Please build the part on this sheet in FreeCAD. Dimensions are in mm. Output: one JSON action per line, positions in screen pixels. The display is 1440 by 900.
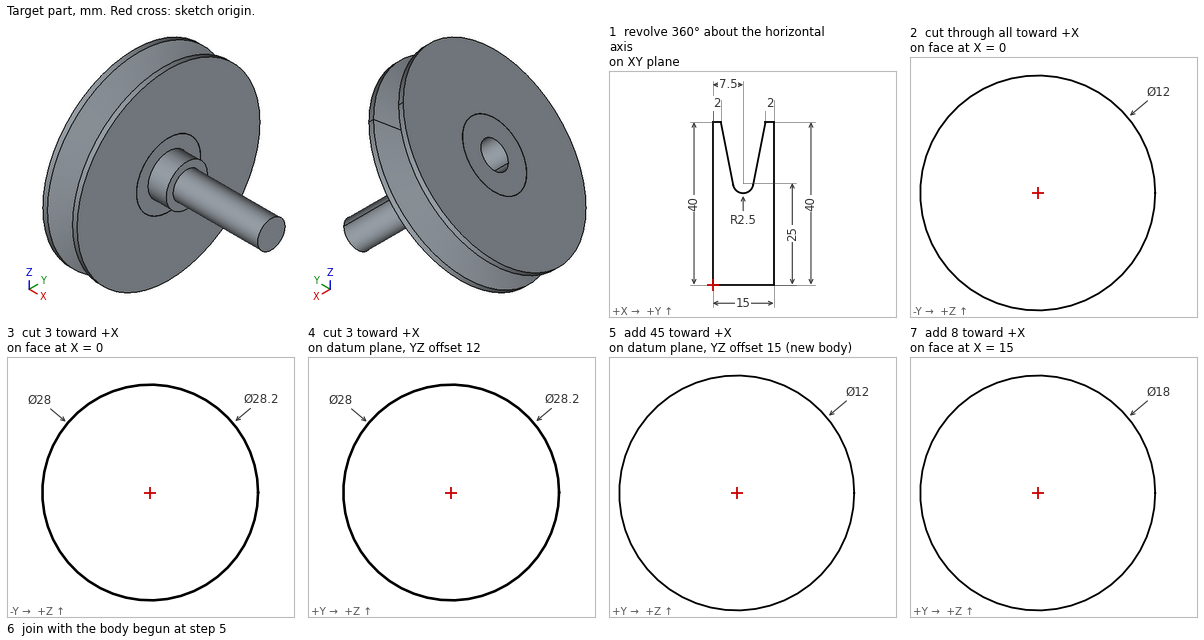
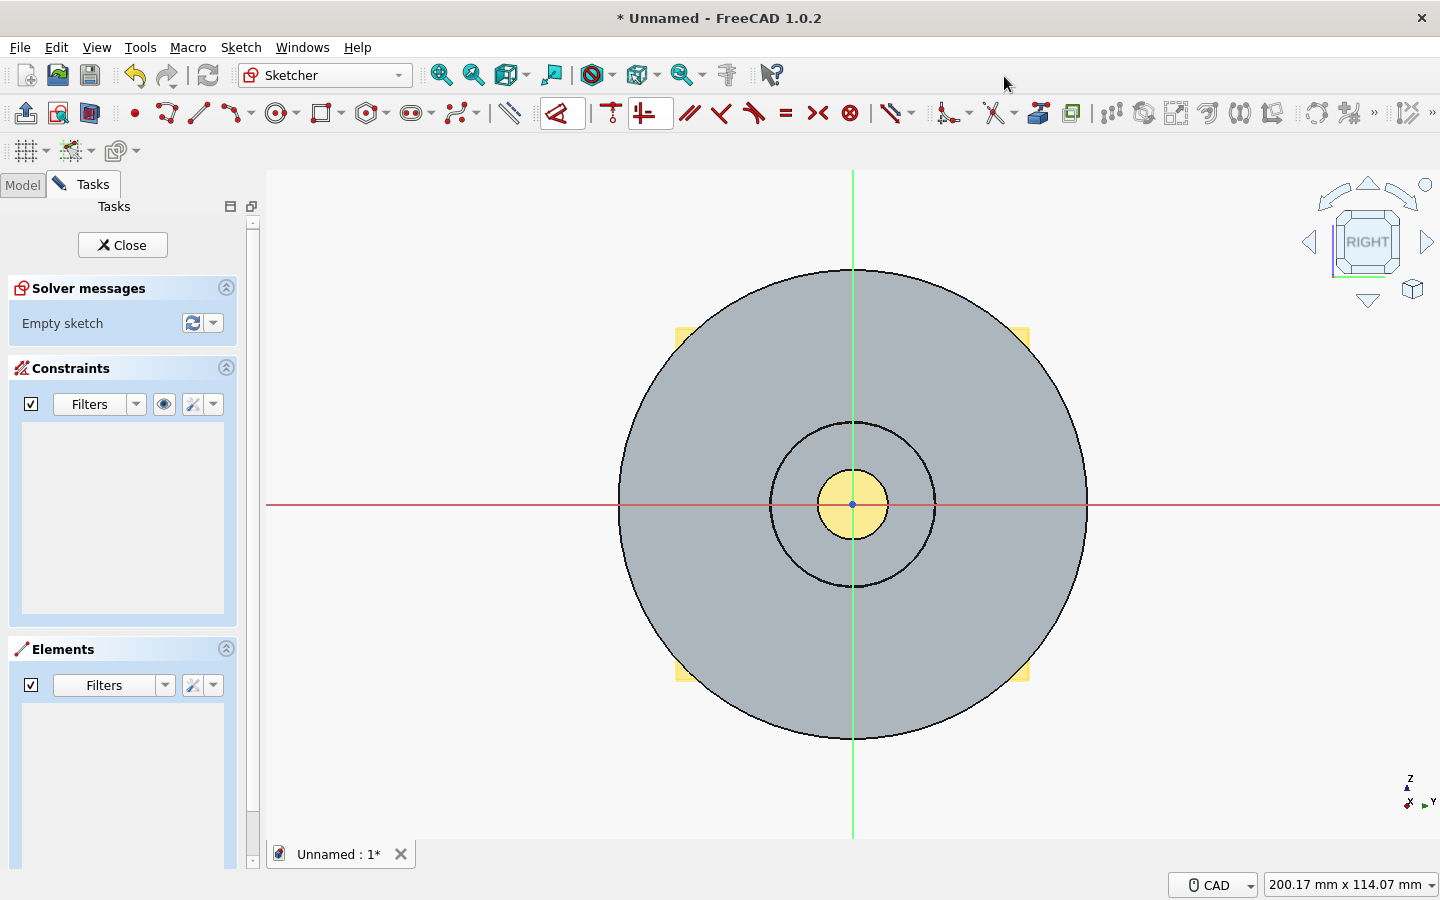
{"action": "scroll", "coordinate": [866, 505], "scroll_direction": "up", "scroll_amount": 9}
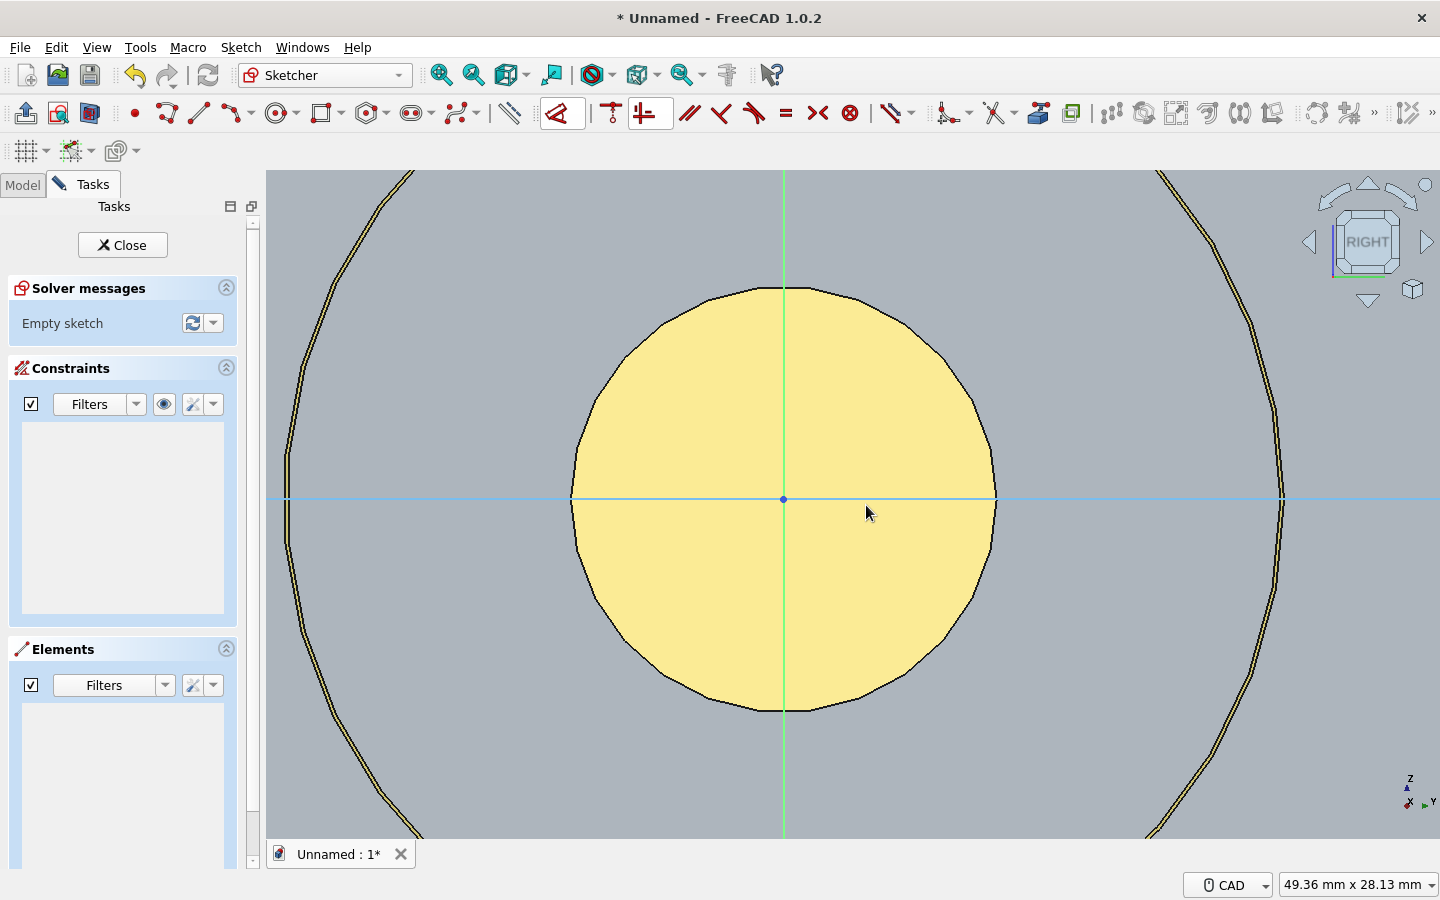
{"action": "left_click", "coordinate": [276, 114]}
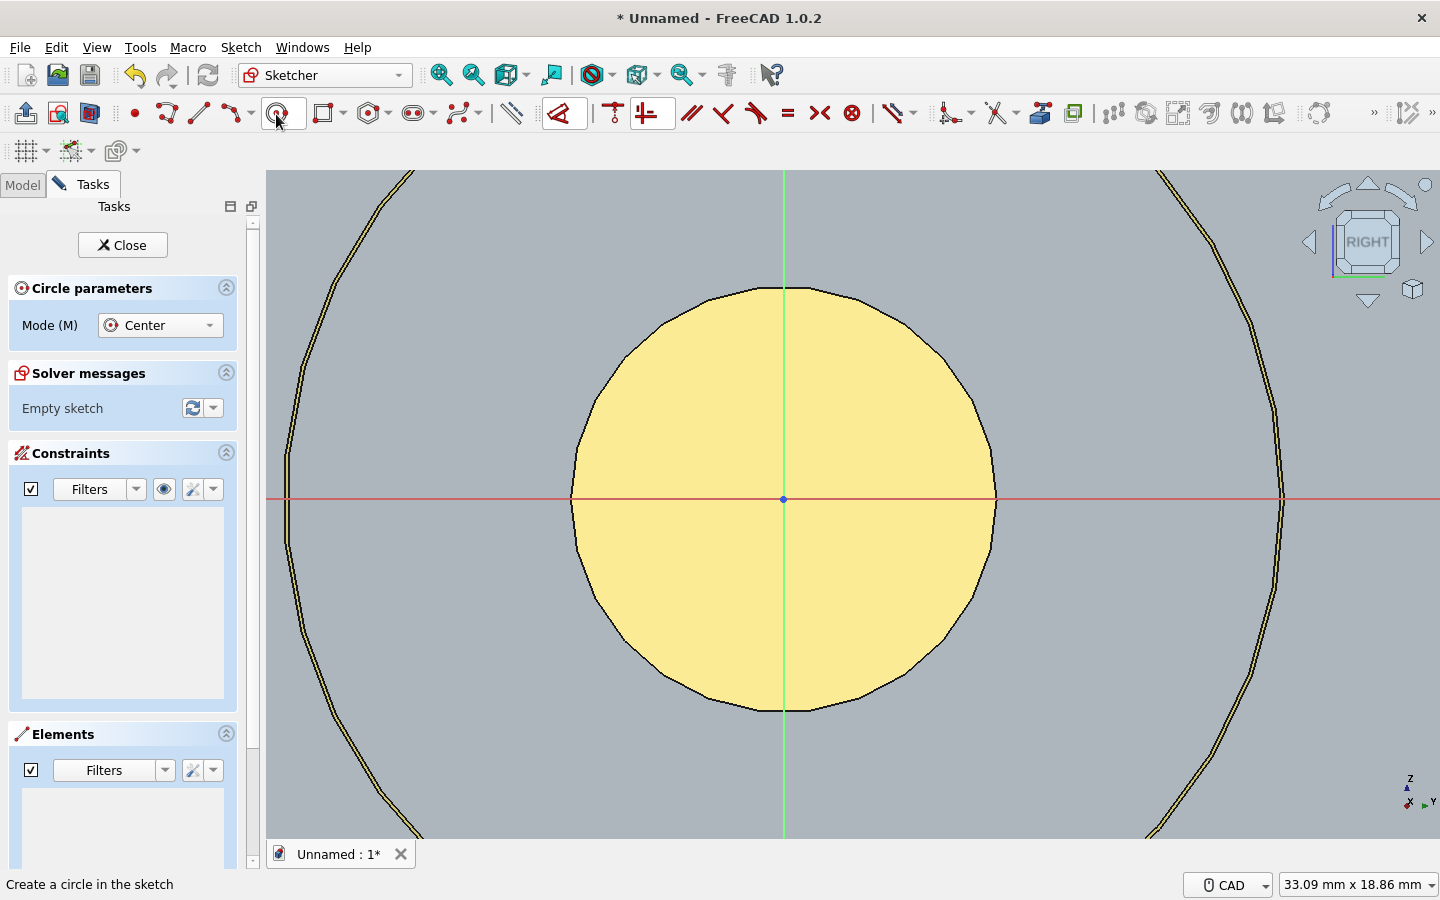
{"action": "left_click", "coordinate": [784, 499]}
{"action": "mouse_move", "coordinate": [934, 349]}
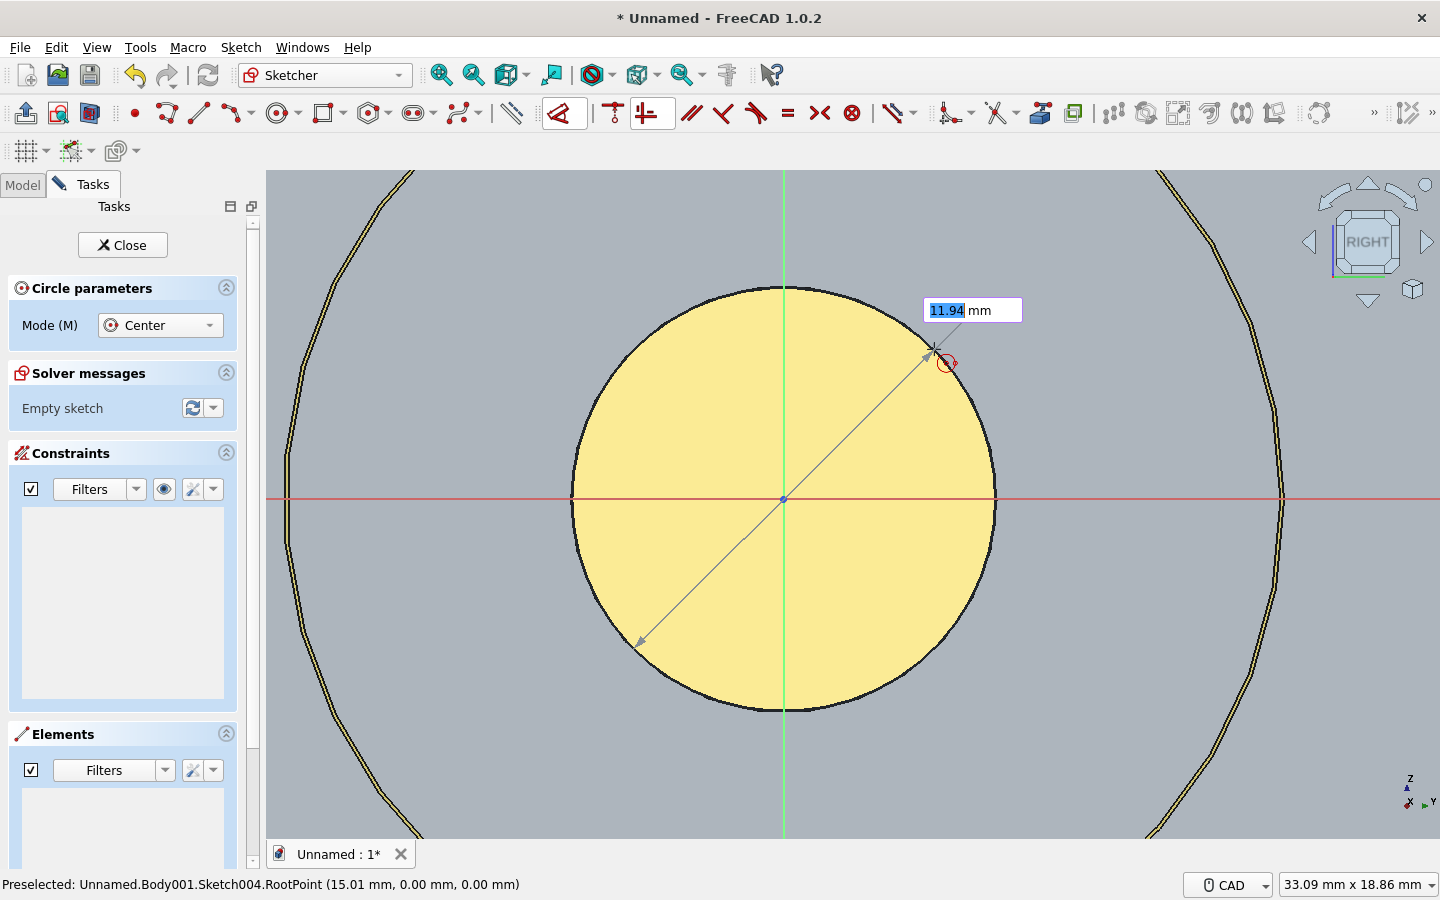
{"action": "type", "text": "12"}
{"action": "key", "text": "Return"}
{"action": "key", "text": "Escape"}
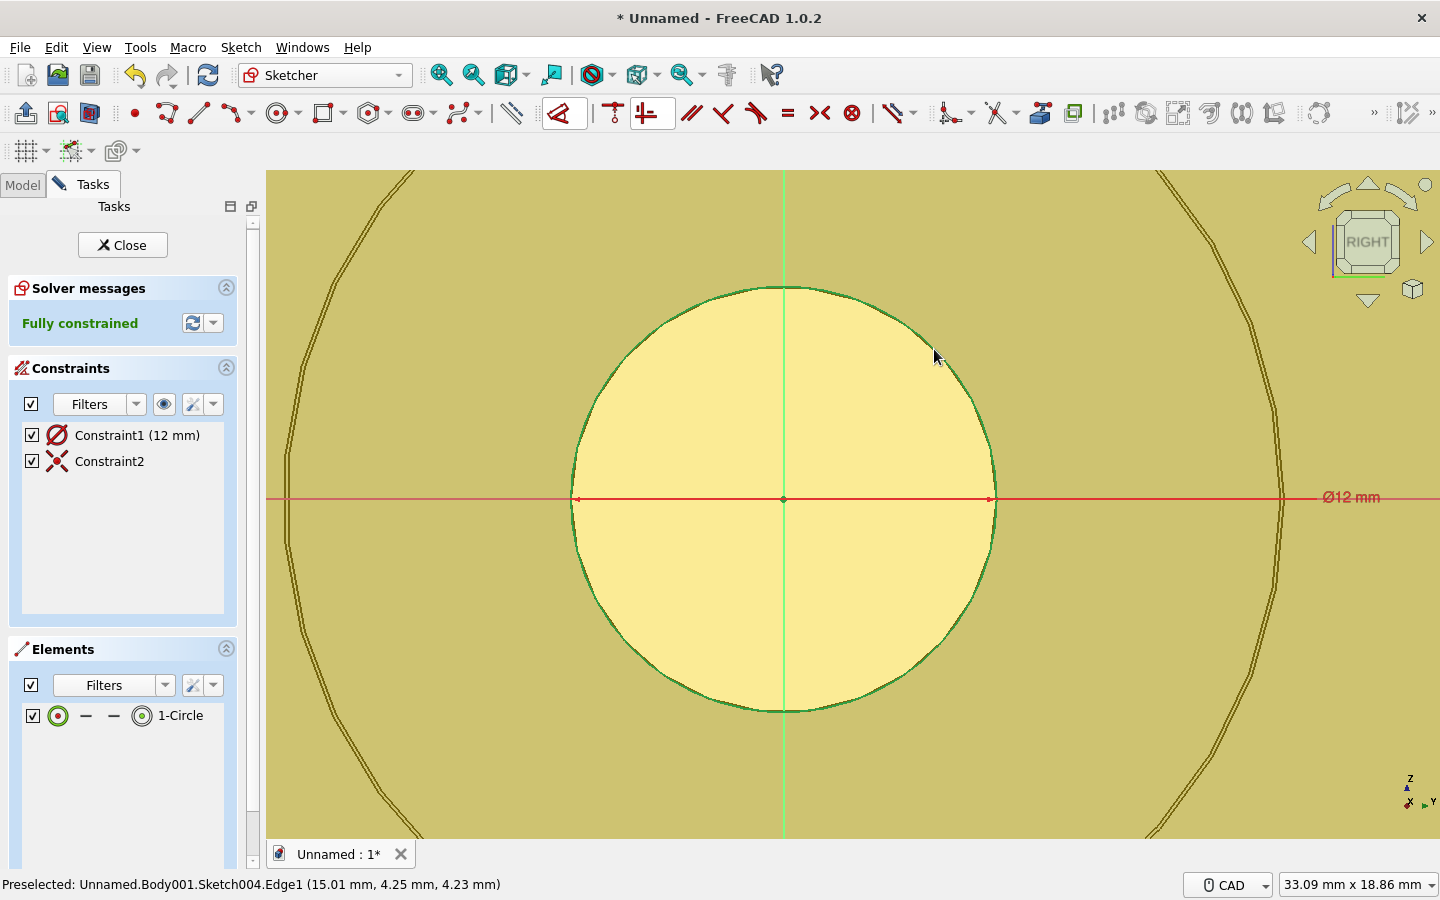
{"action": "left_click", "coordinate": [123, 245]}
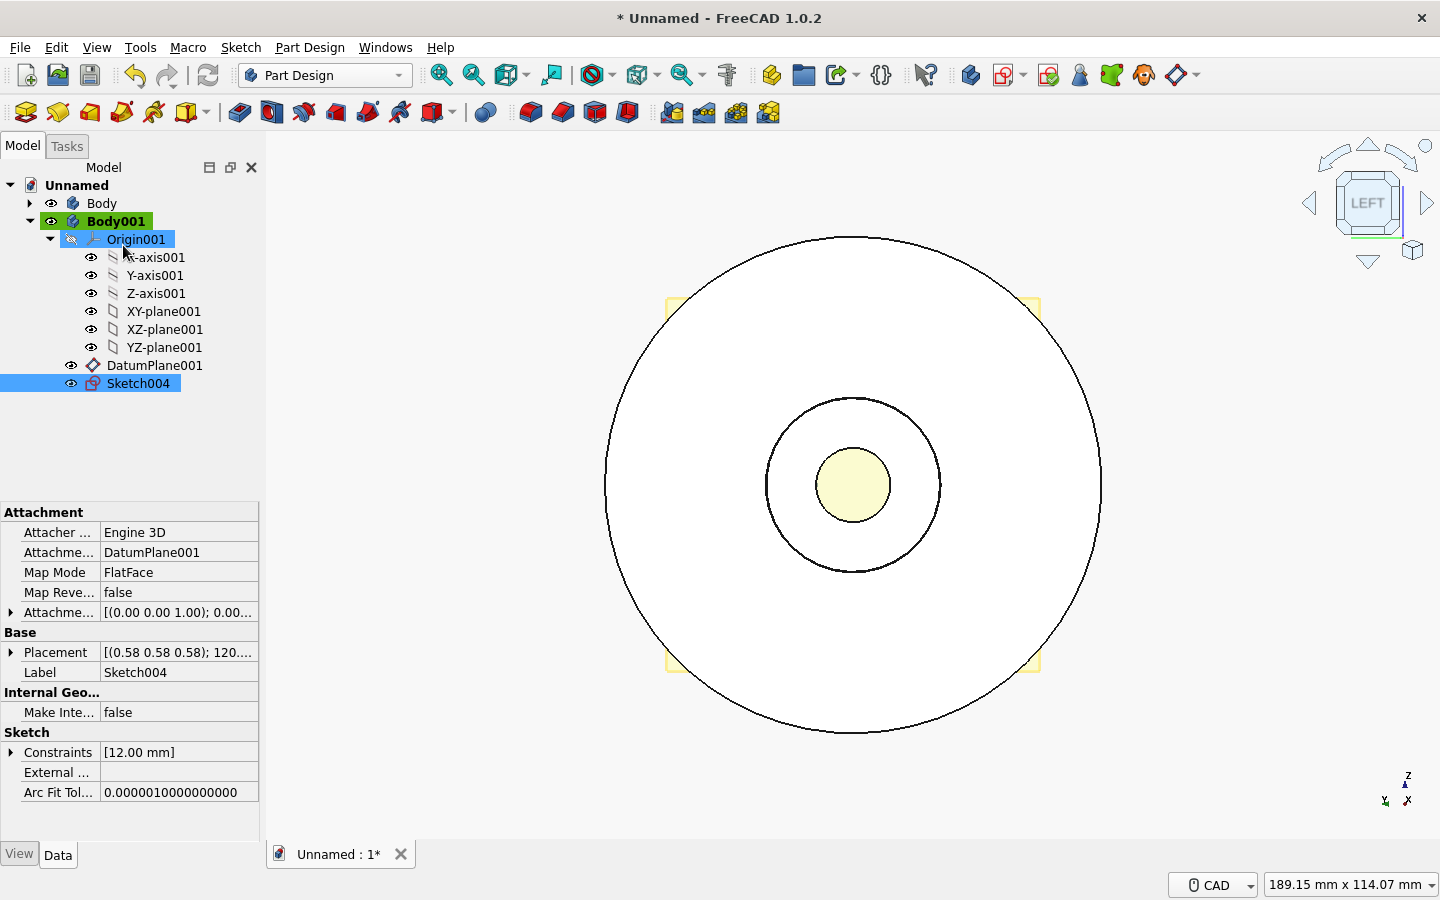
{"action": "left_click", "coordinate": [26, 112]}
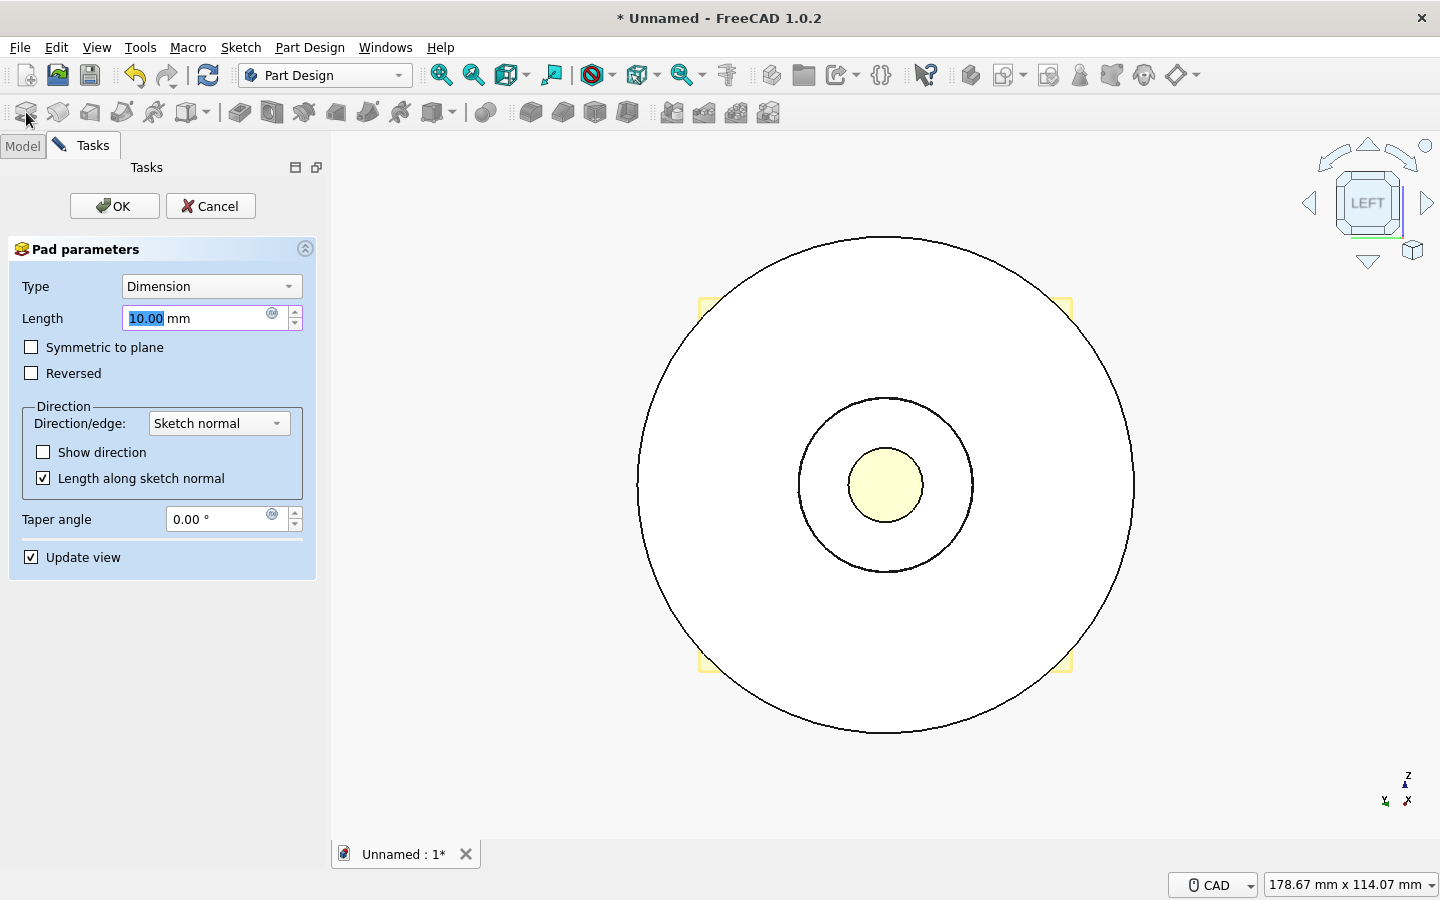
{"action": "type", "text": "45"}
{"action": "key", "text": "Tab"}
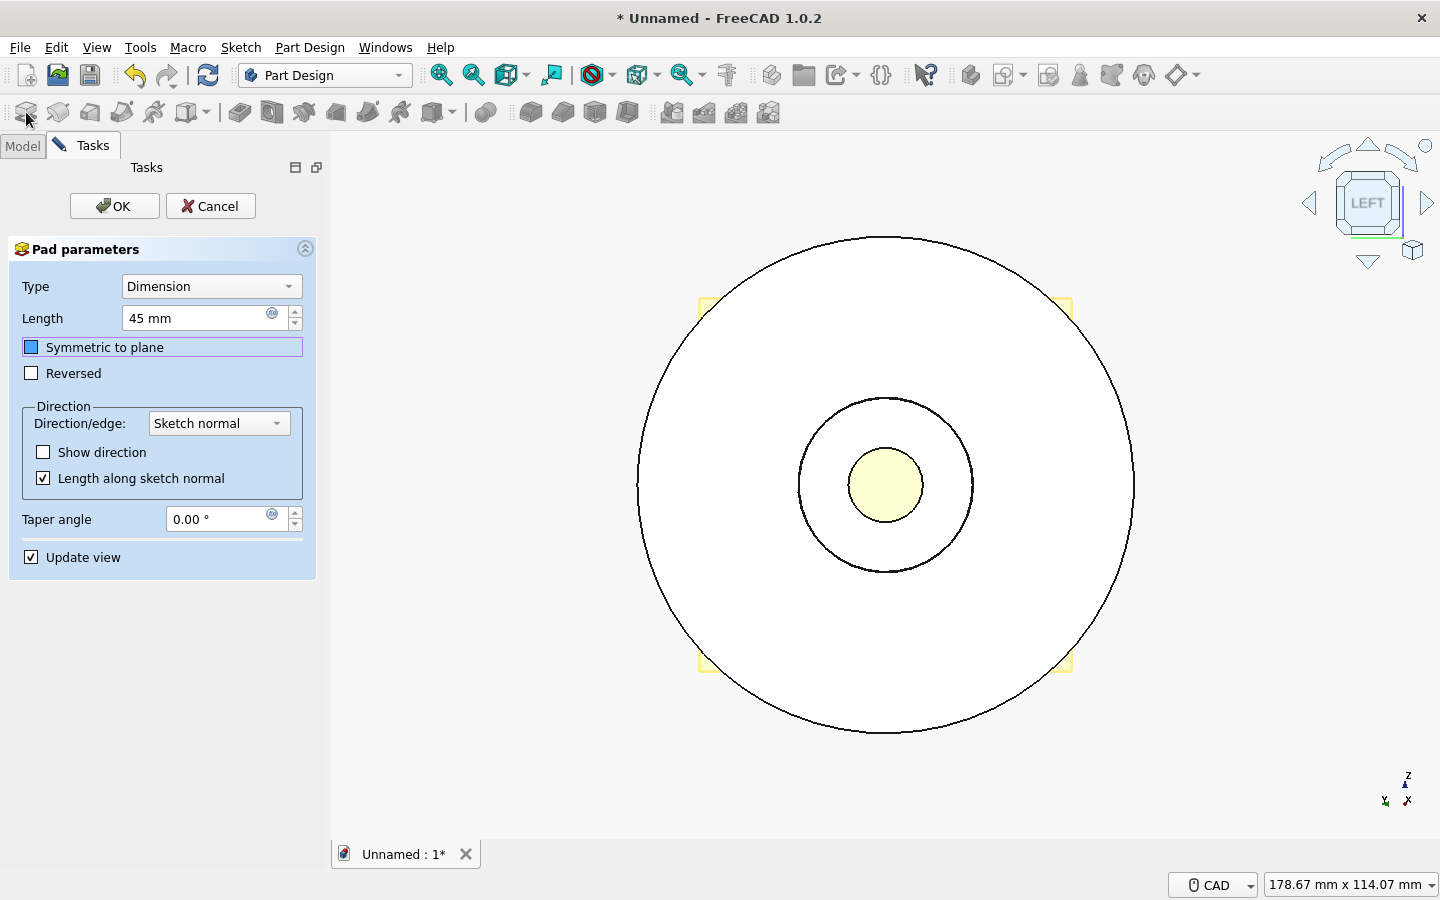
{"action": "left_click", "coordinate": [115, 206]}